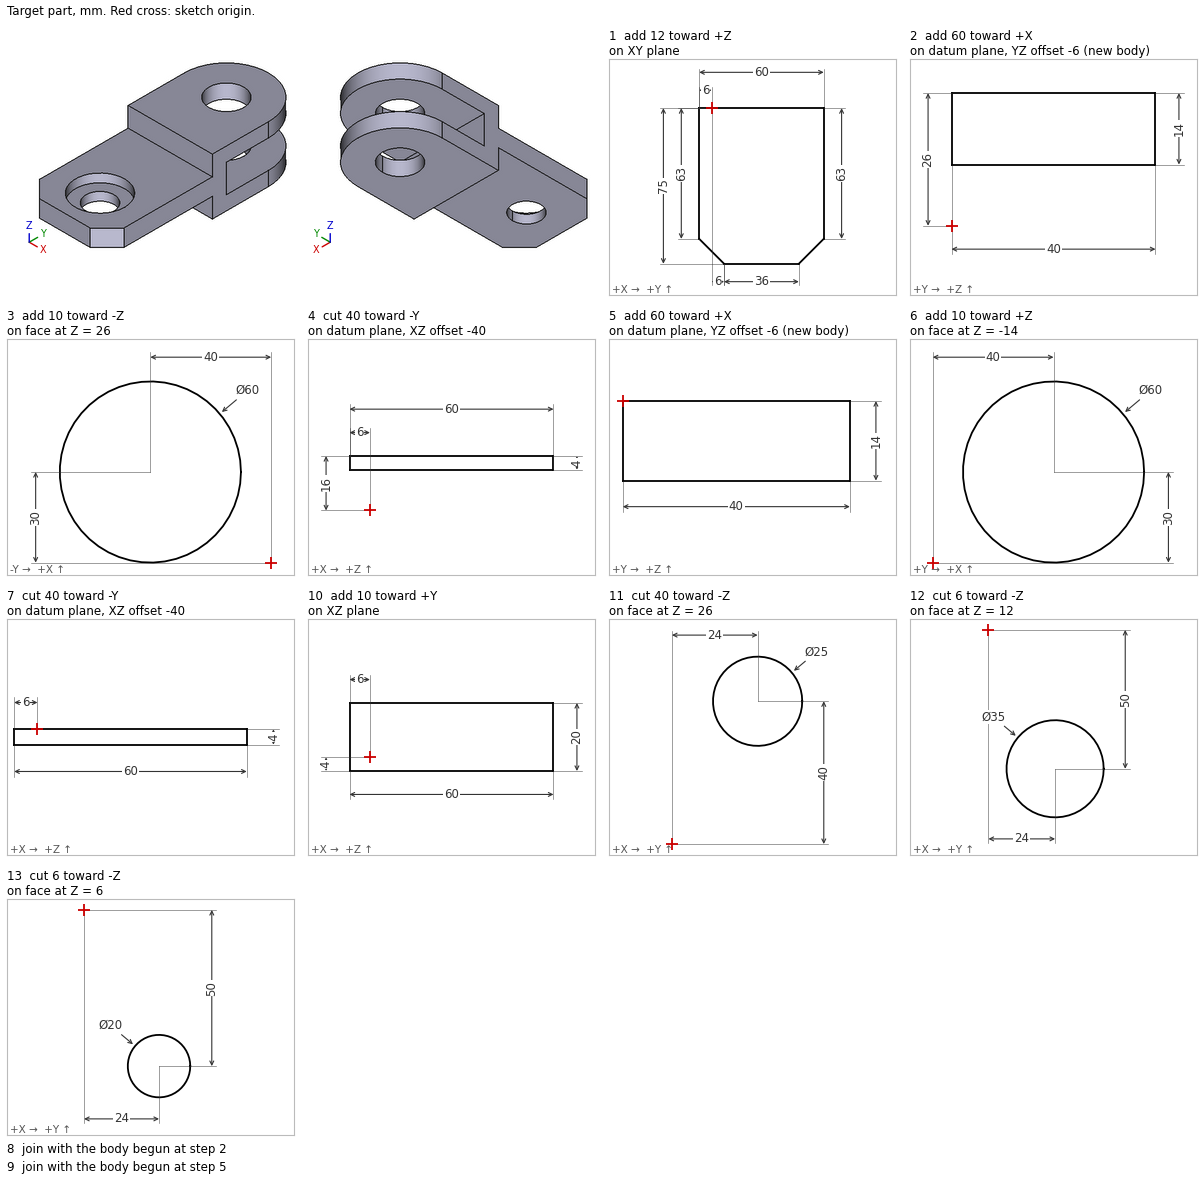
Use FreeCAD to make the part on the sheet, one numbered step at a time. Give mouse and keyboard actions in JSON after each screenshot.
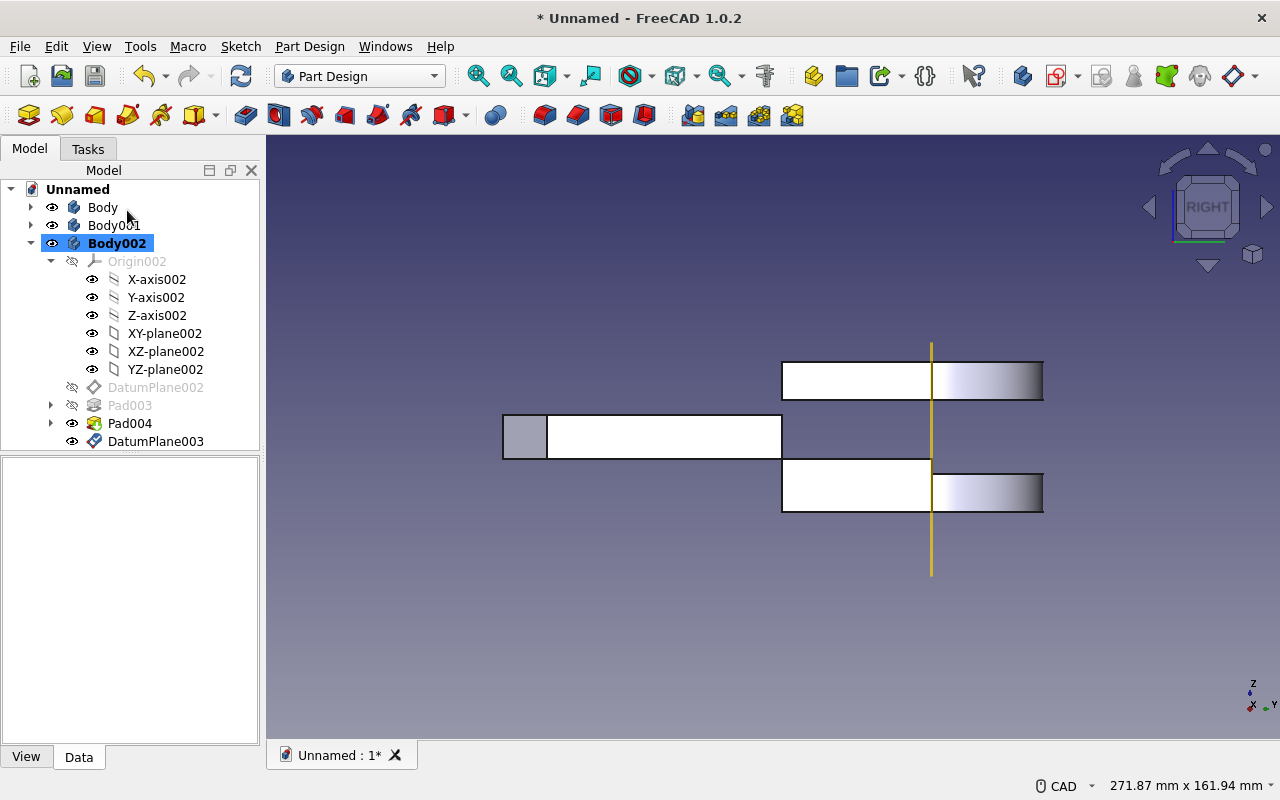
{"action": "left_click", "coordinate": [117, 441]}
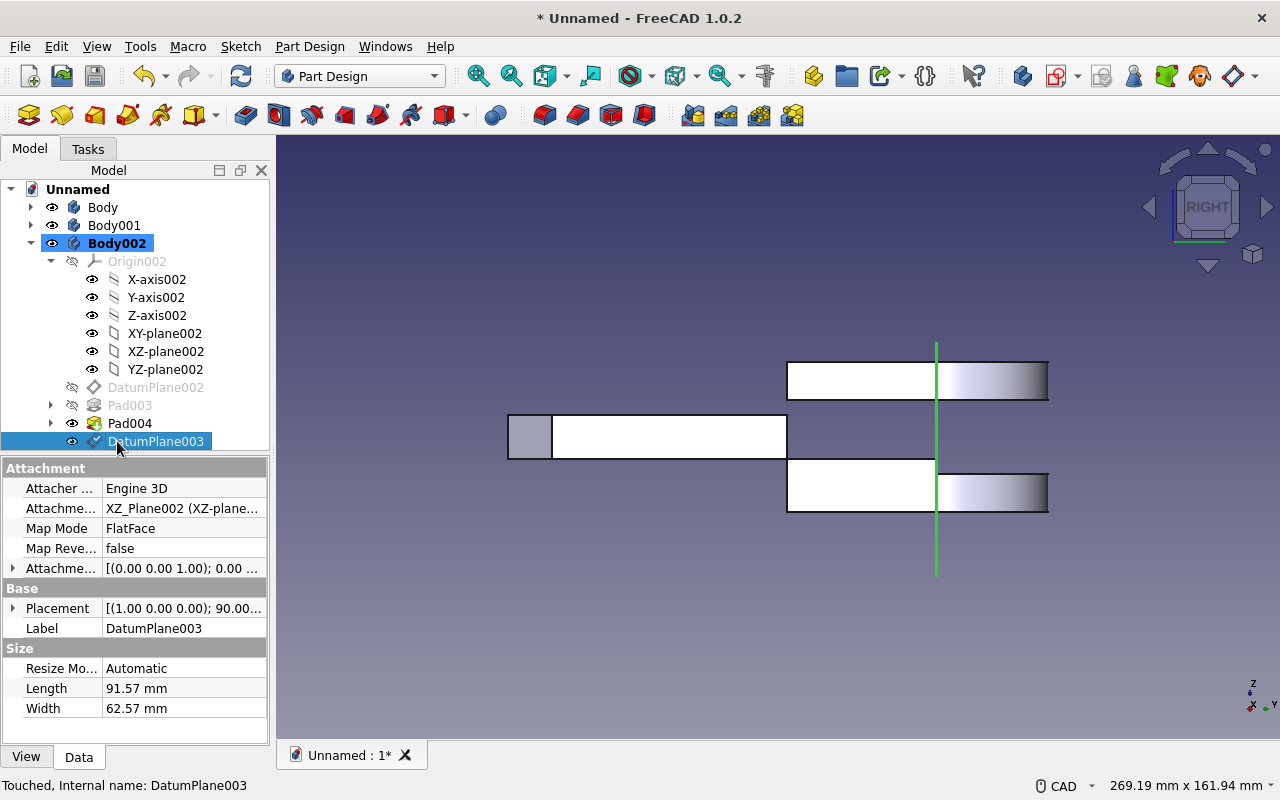
{"action": "left_click", "coordinate": [1056, 76]}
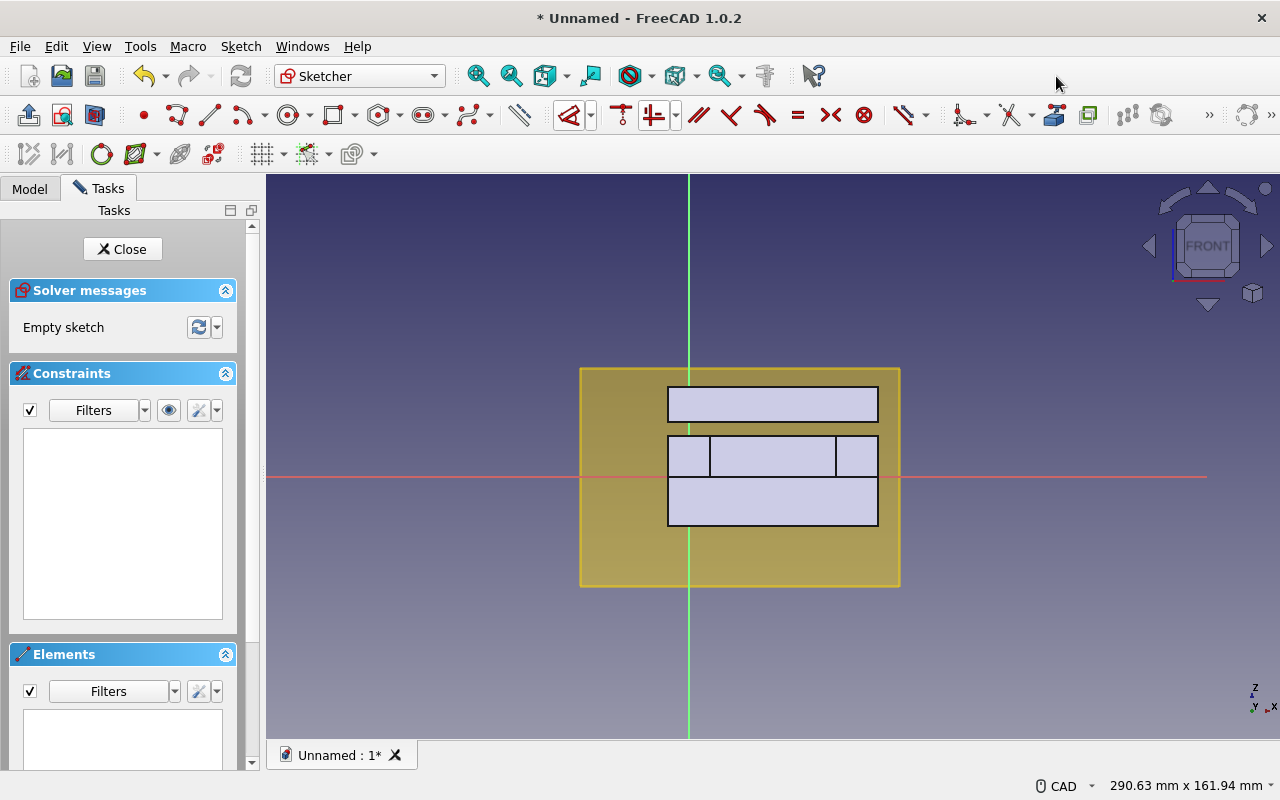
{"action": "key", "text": "q s"}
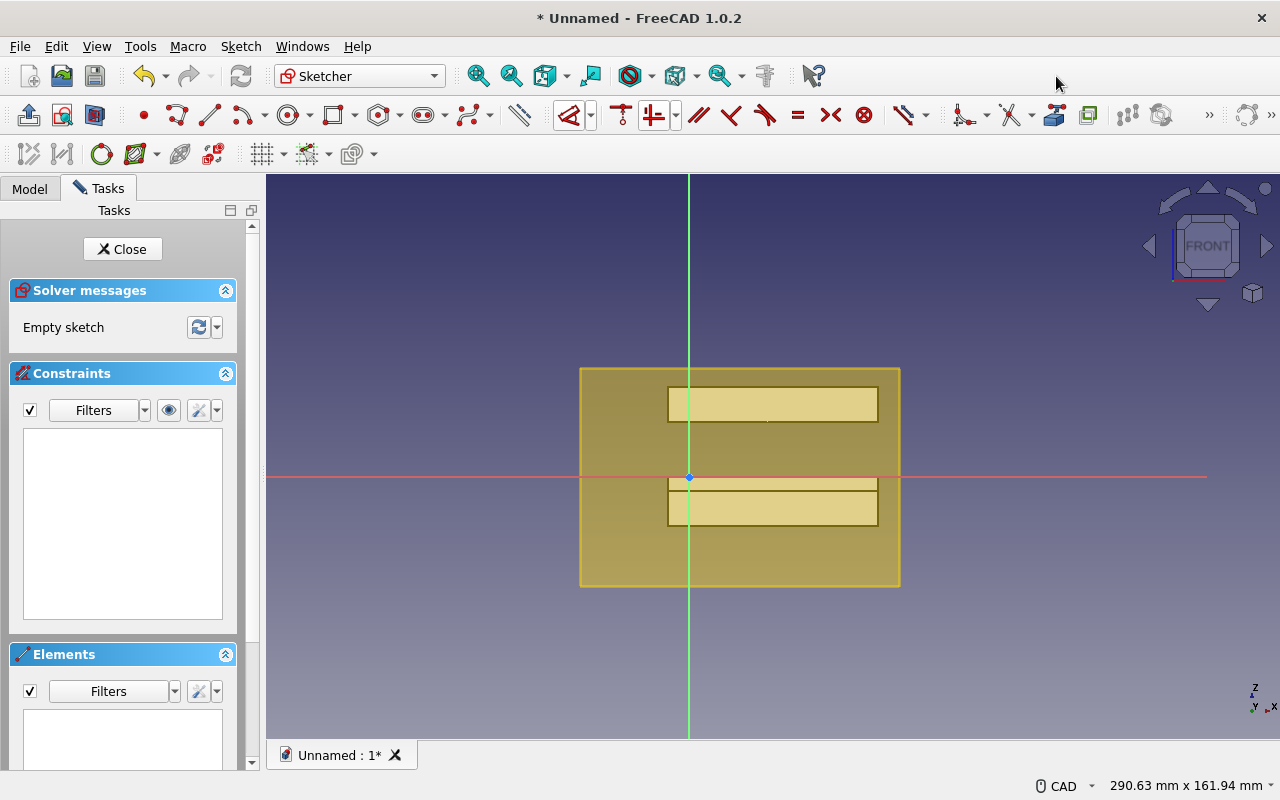
{"action": "scroll", "coordinate": [813, 501], "scroll_direction": "up", "scroll_amount": 5}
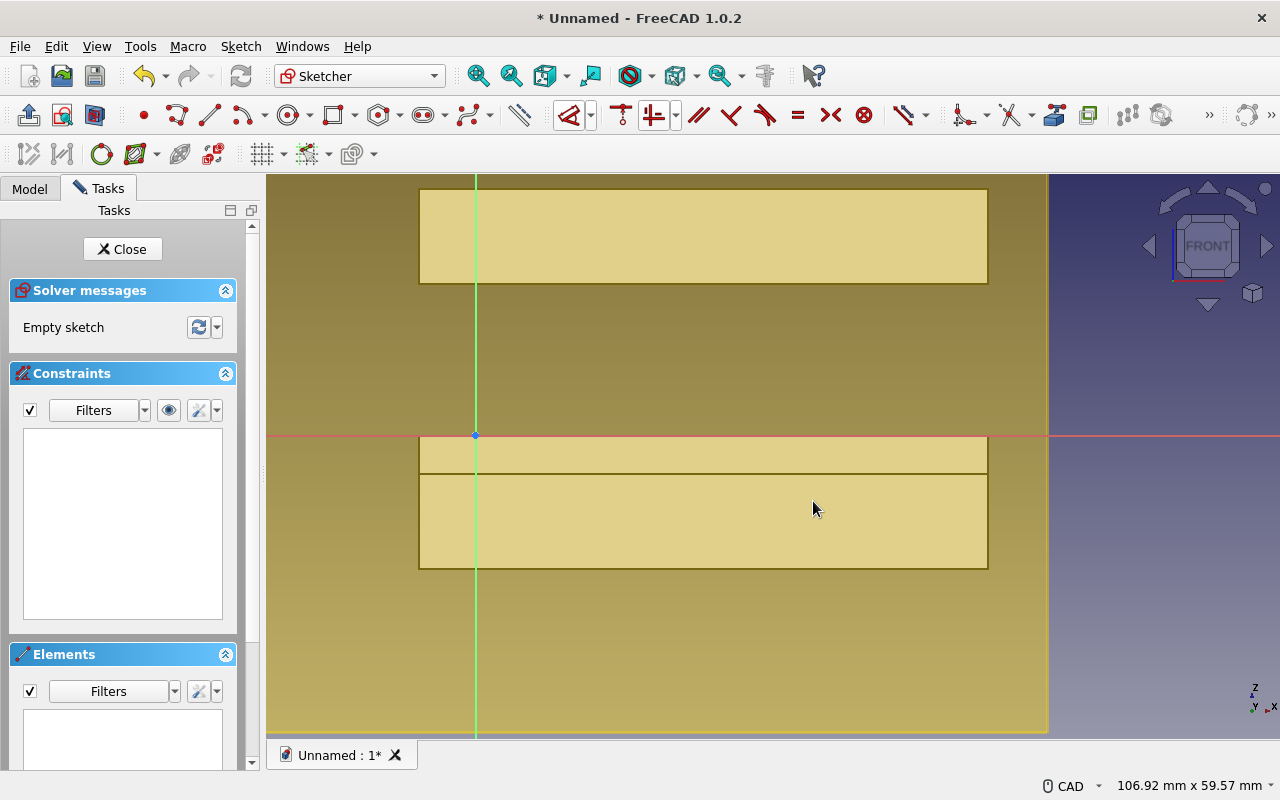
{"action": "left_click", "coordinate": [332, 116]}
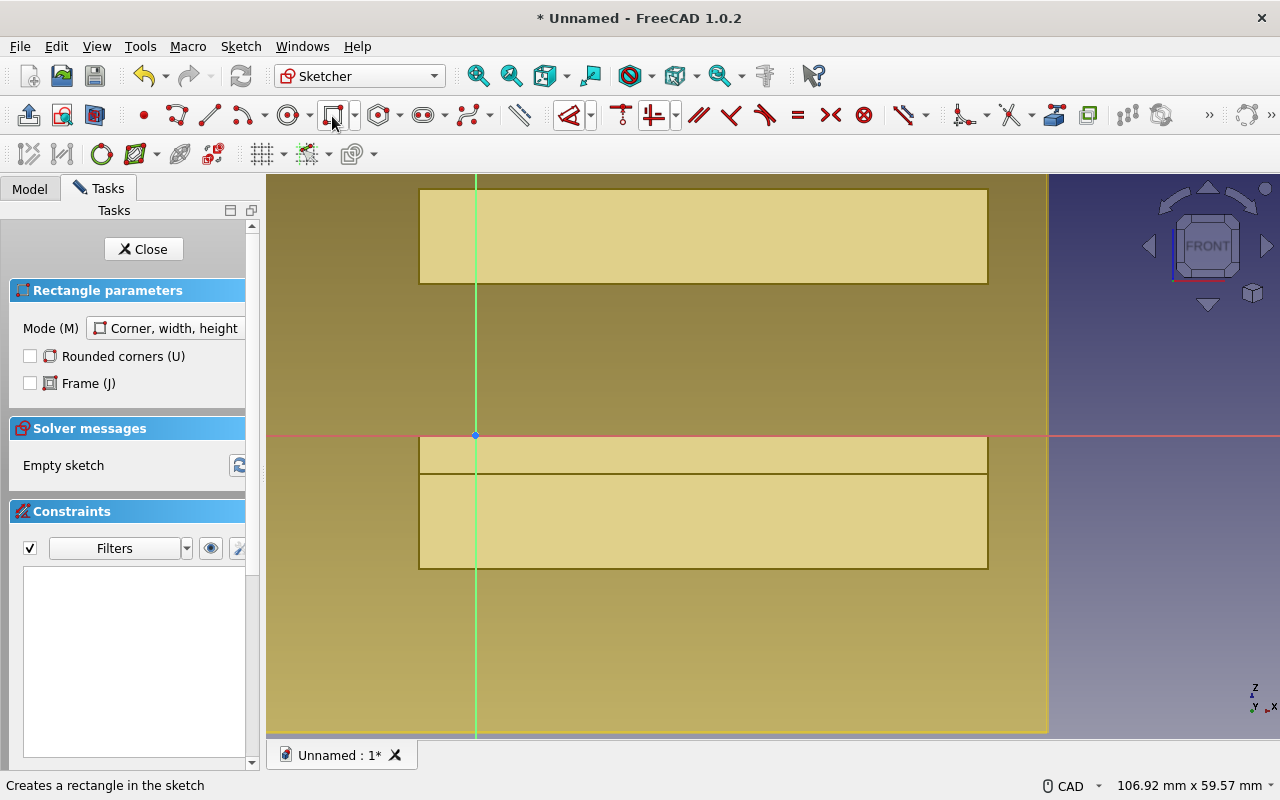
{"action": "left_click", "coordinate": [419, 436]}
{"action": "mouse_move", "coordinate": [988, 474]}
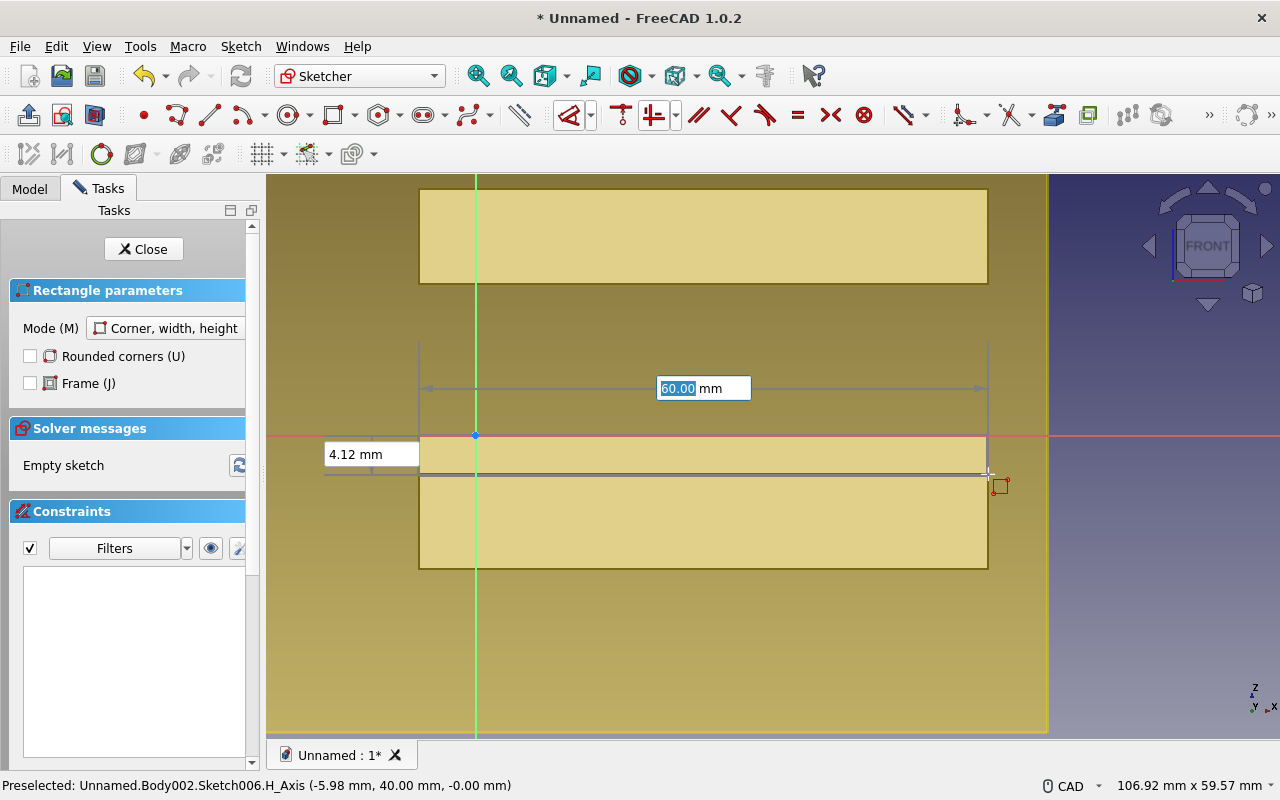
{"action": "type", "text": "60"}
{"action": "key", "text": "Tab"}
{"action": "type", "text": "4"}
{"action": "key", "text": "Return"}
{"action": "key", "text": "Escape"}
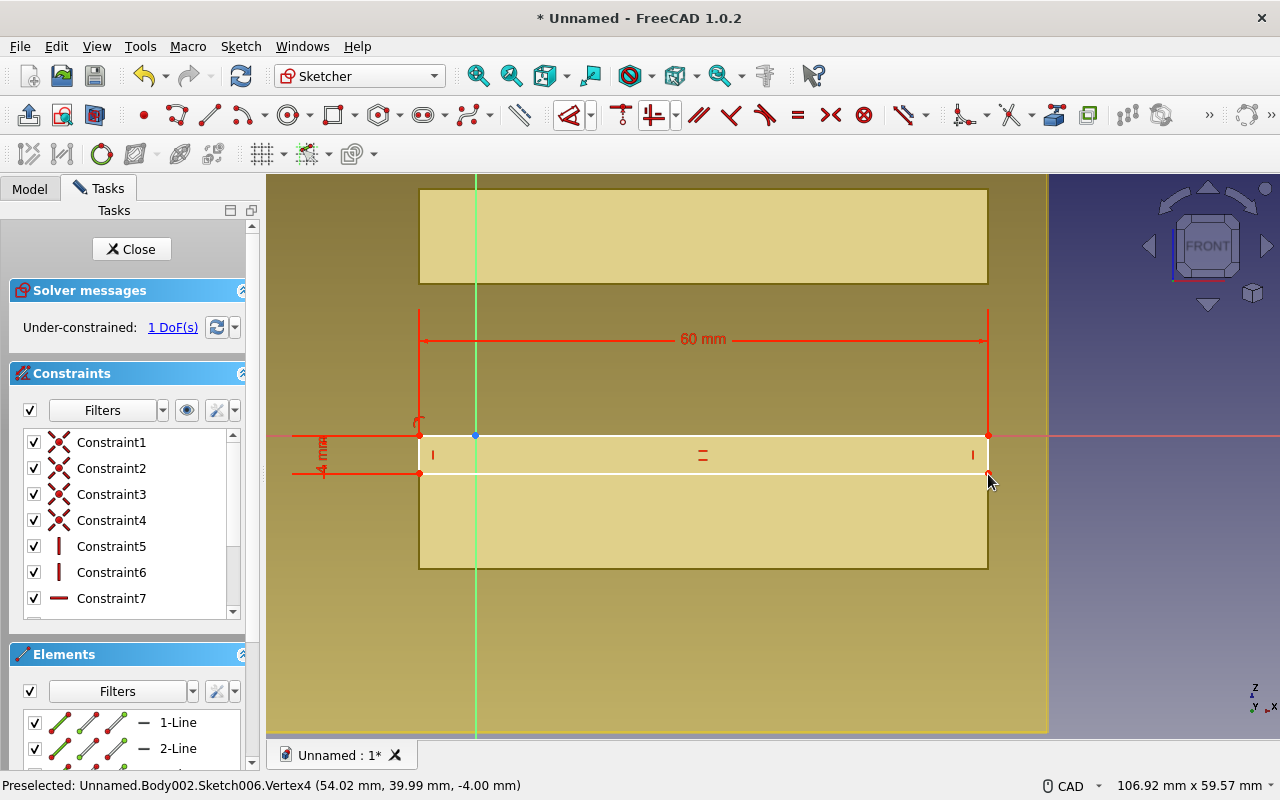
{"action": "left_click", "coordinate": [419, 436]}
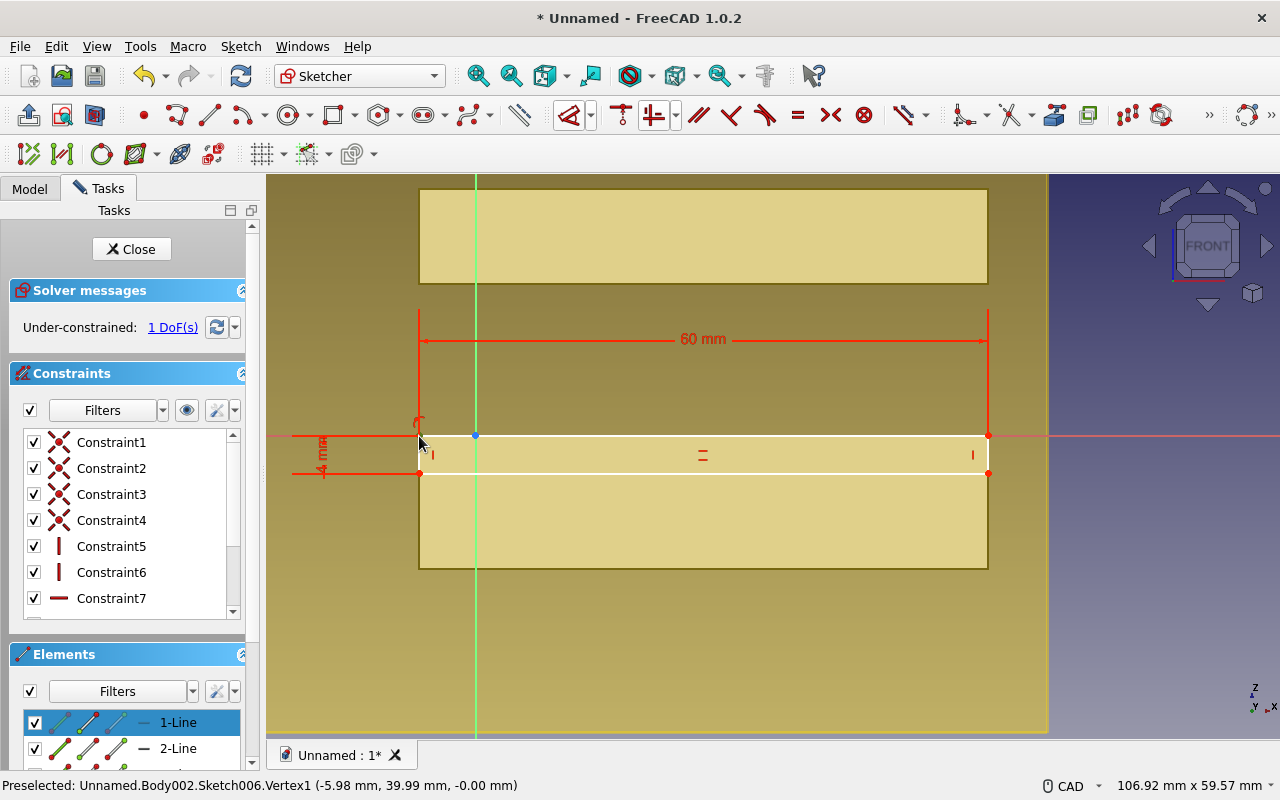
{"action": "key", "text": "l"}